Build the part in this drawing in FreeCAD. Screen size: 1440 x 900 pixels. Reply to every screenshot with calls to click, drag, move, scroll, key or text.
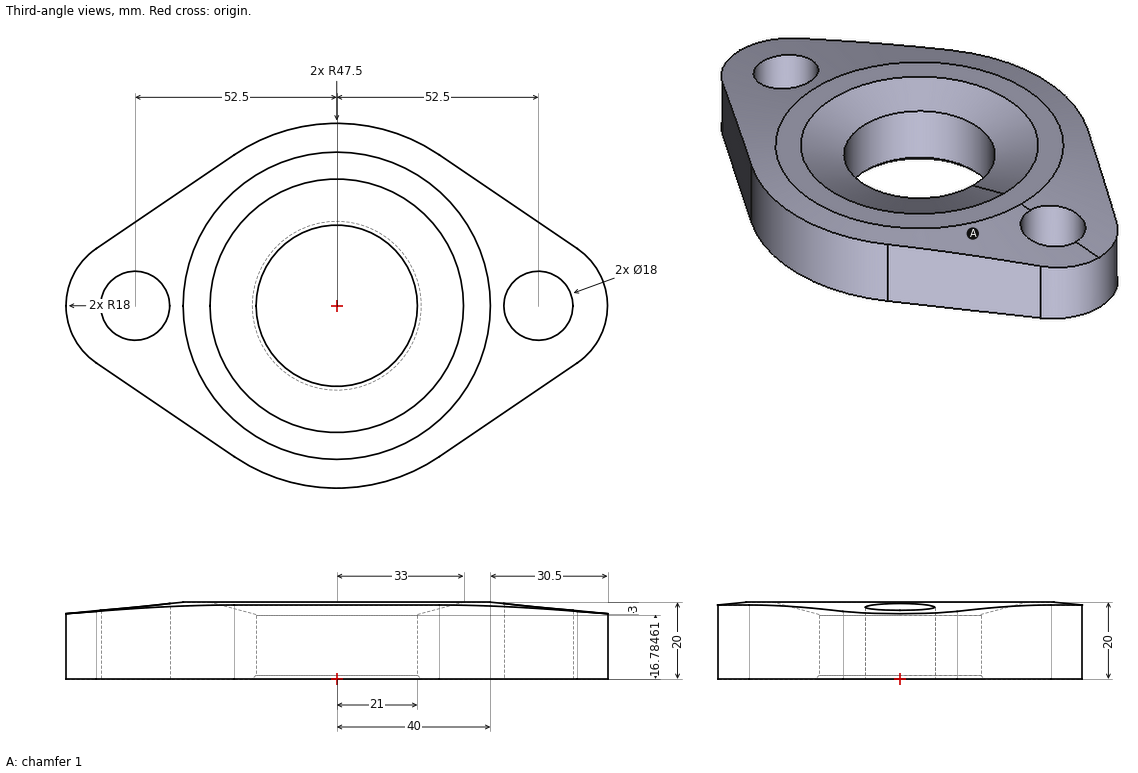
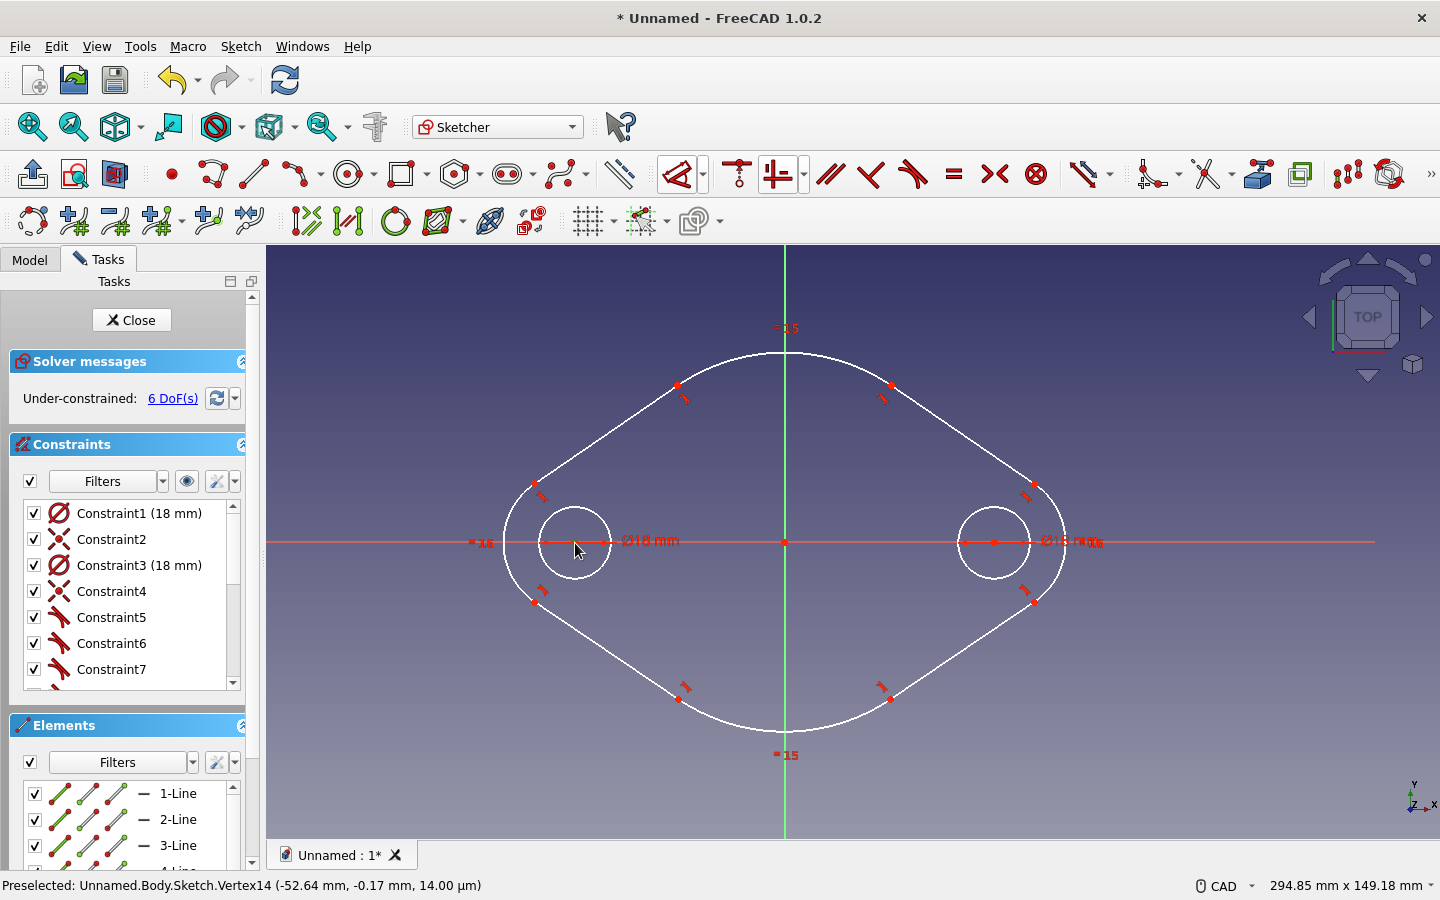
click(364, 542)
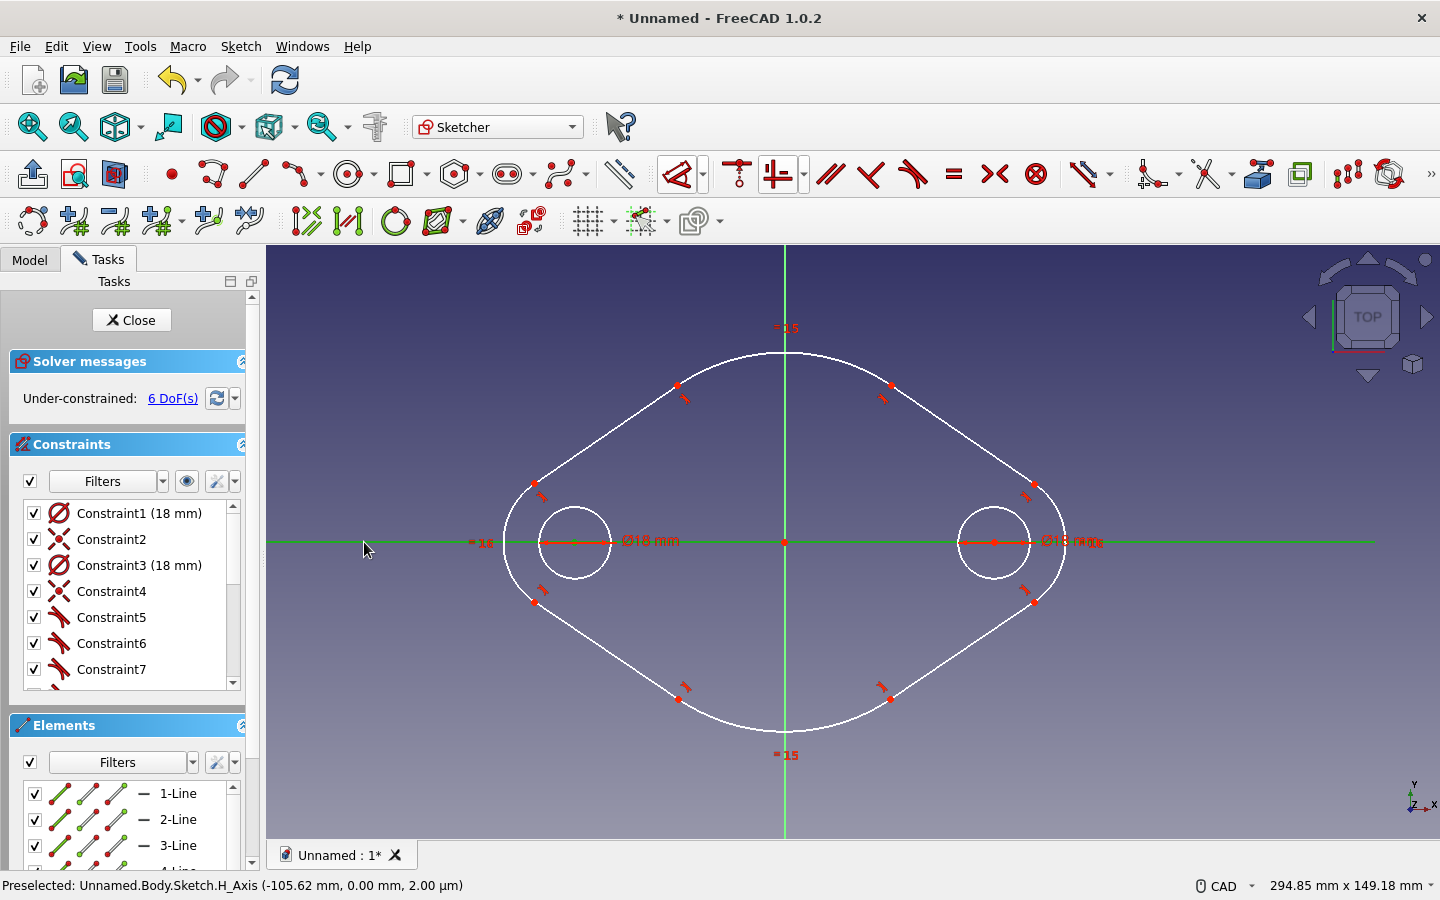
click(737, 174)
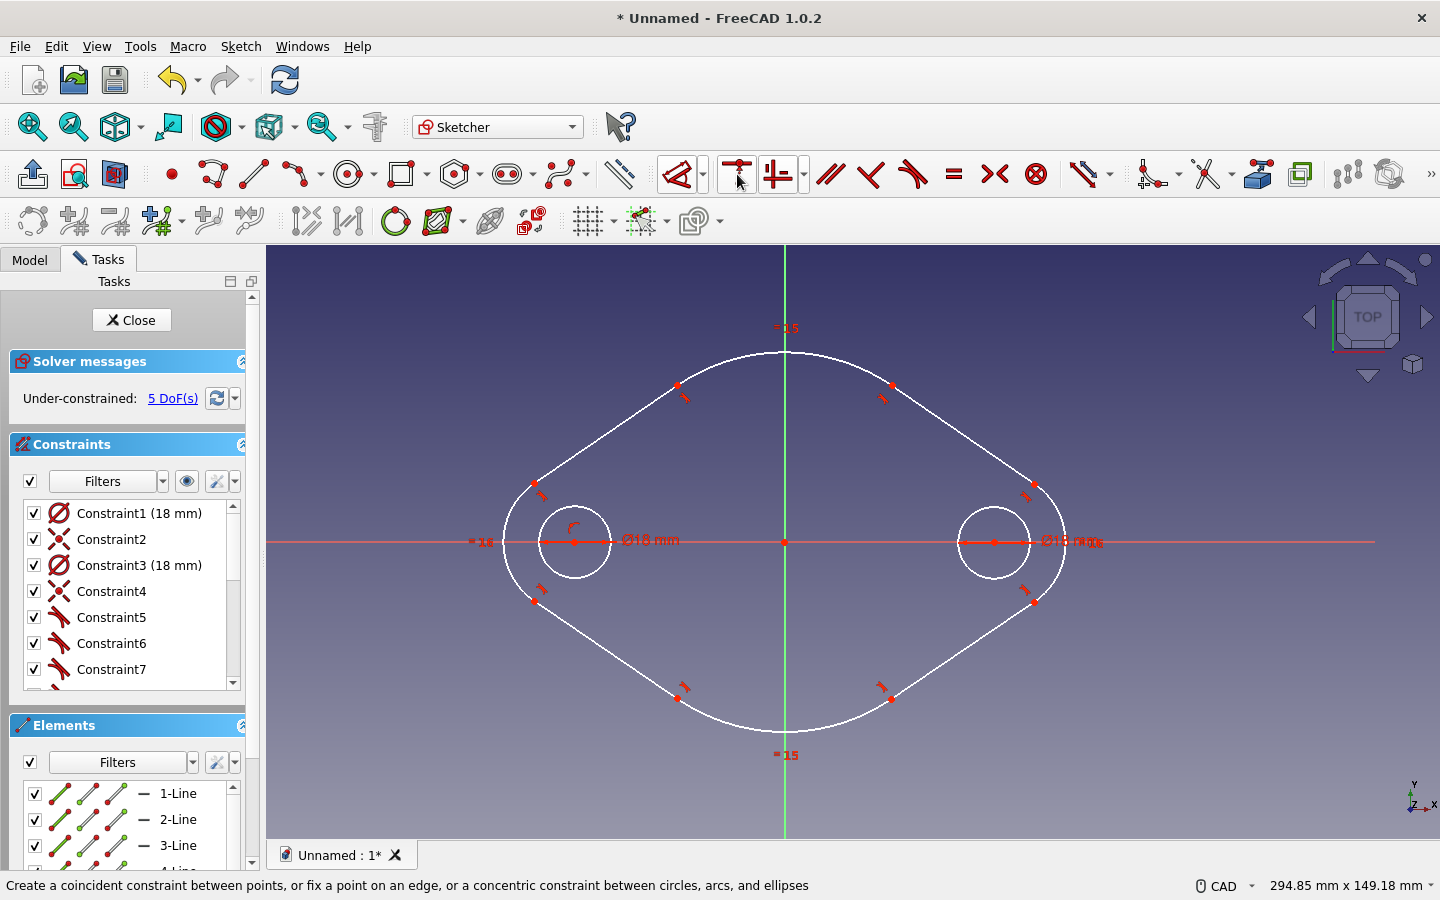
click(994, 543)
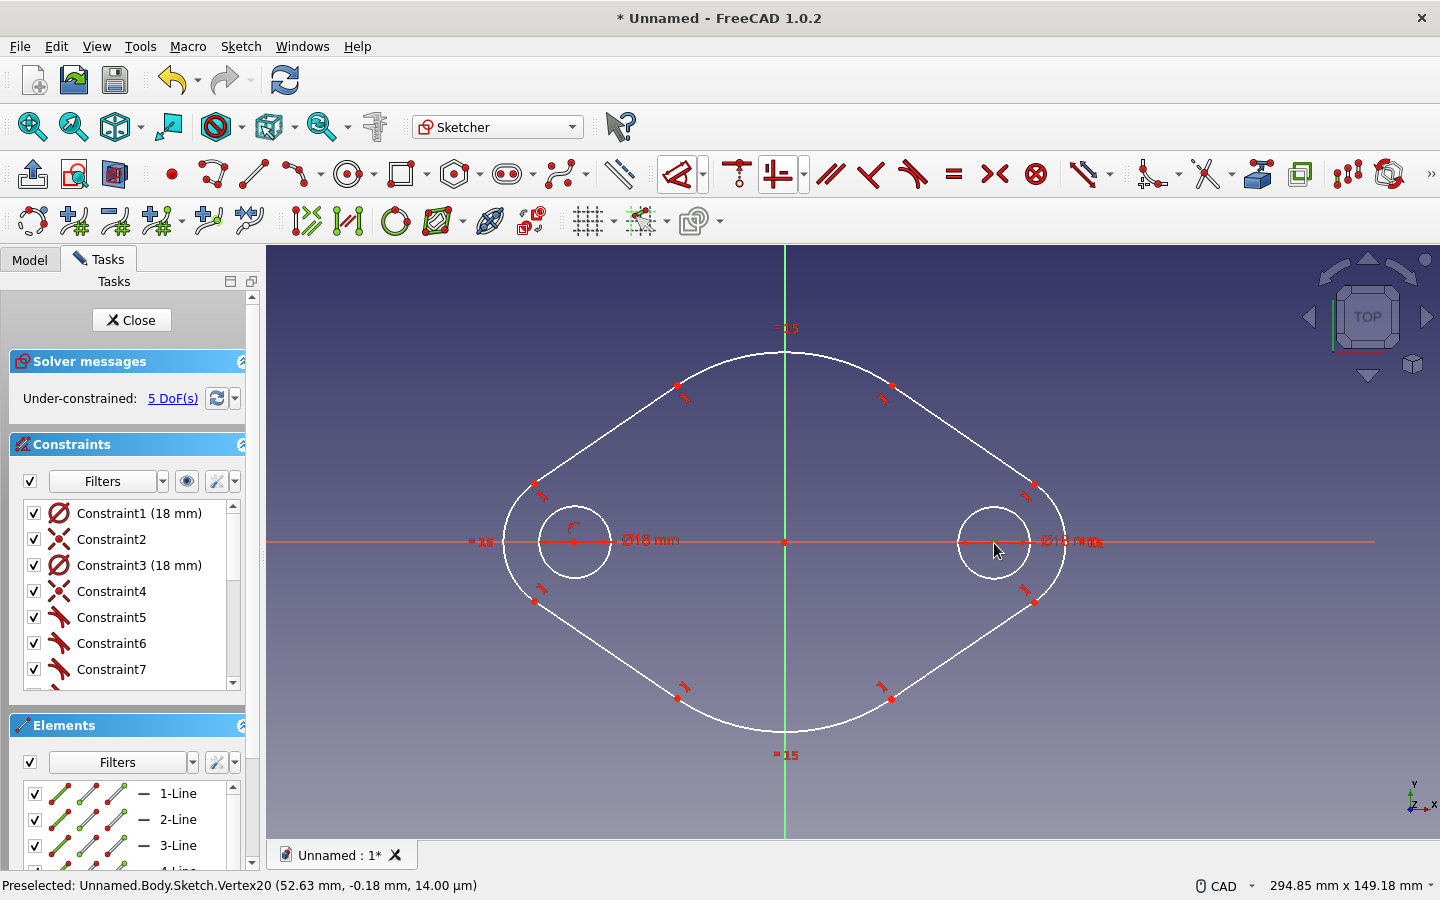
click(364, 542)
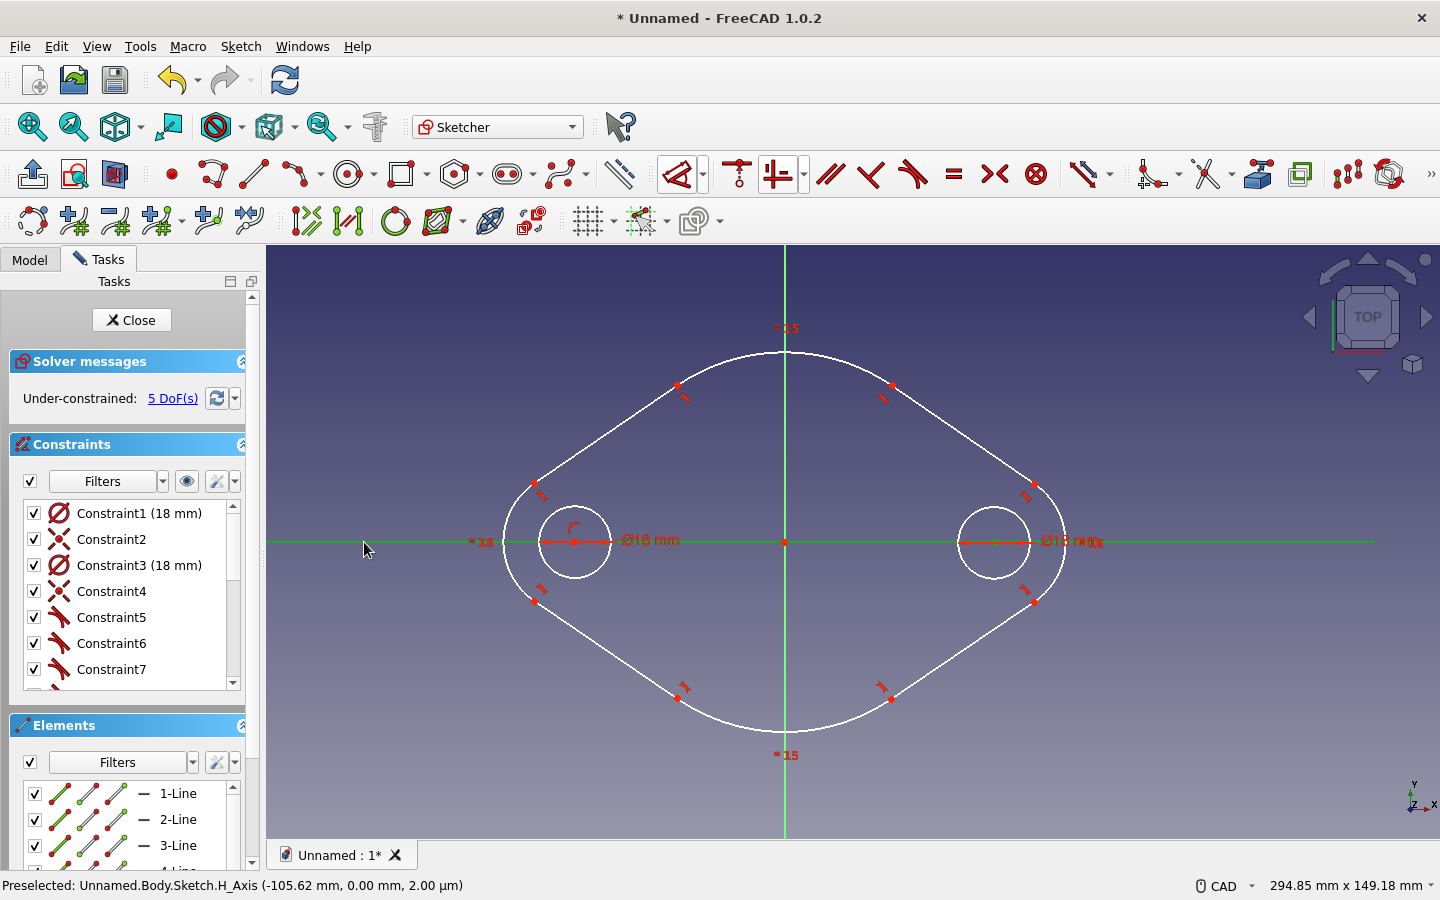
key(c)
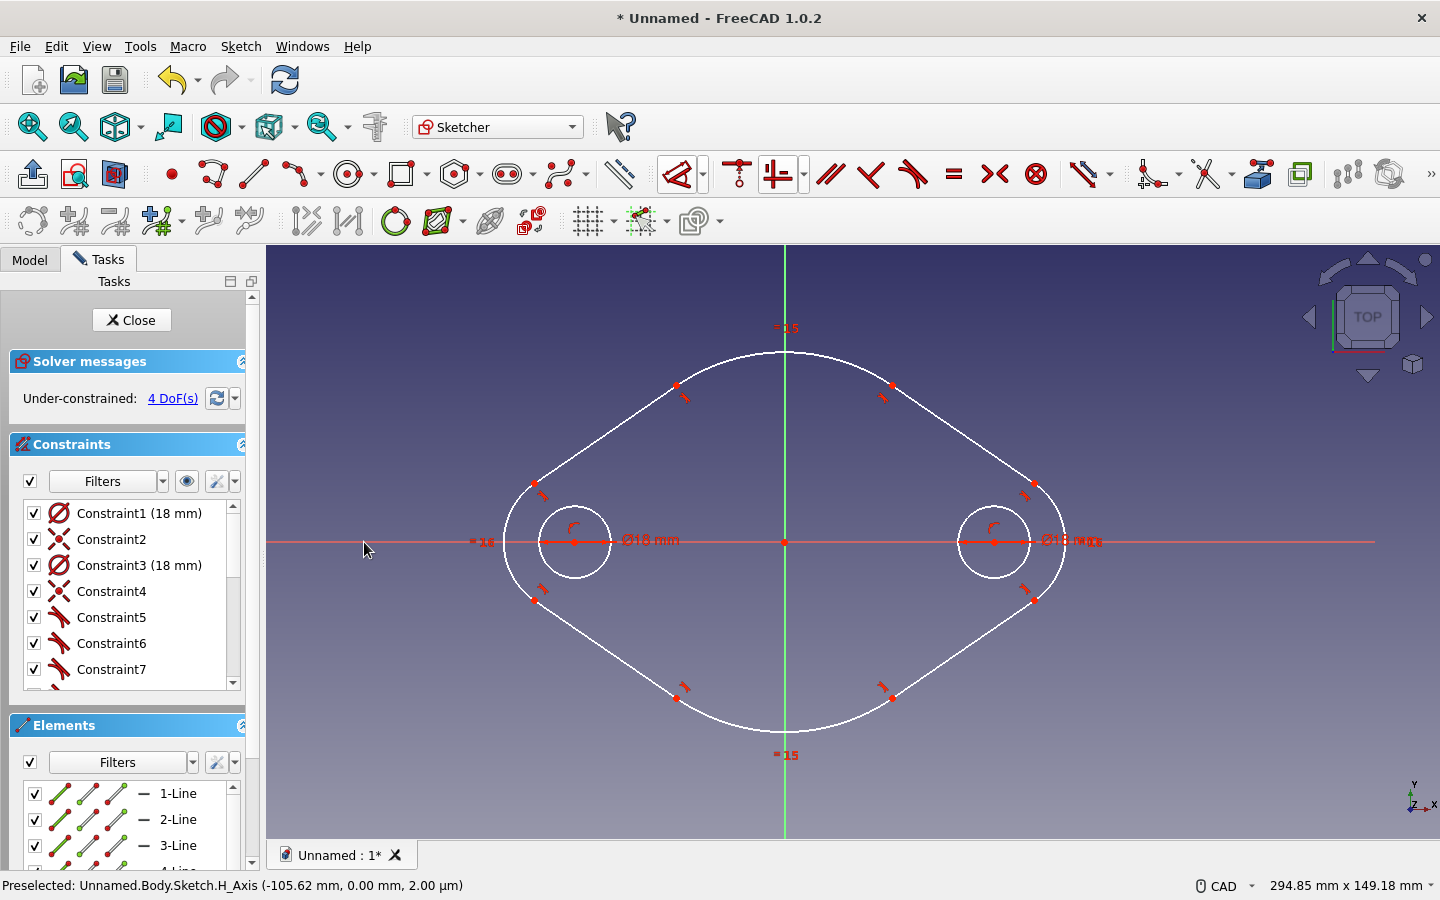
key(d)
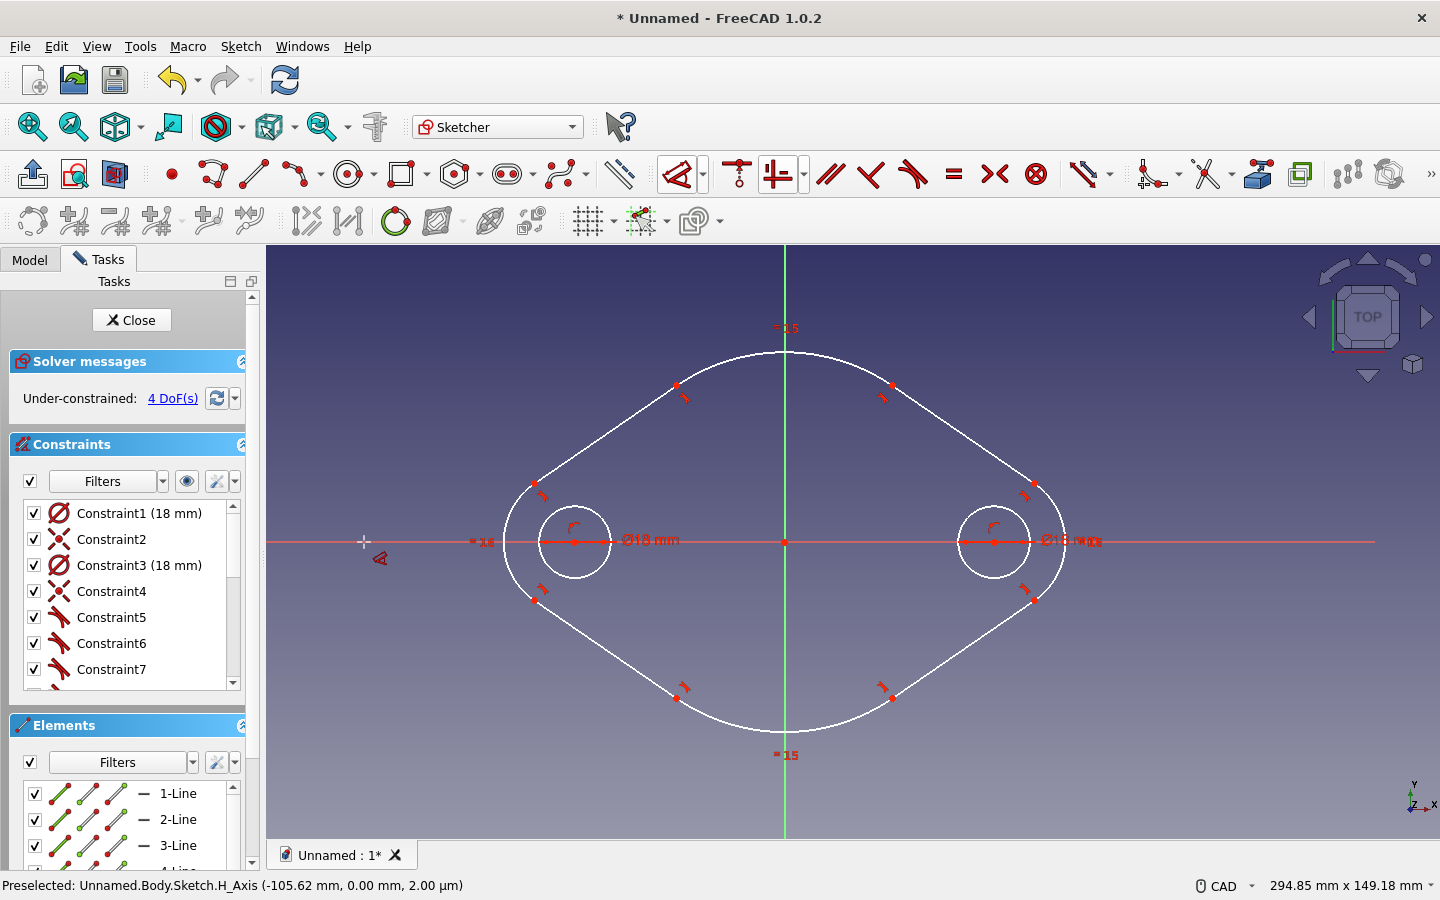
click(830, 358)
click(838, 327)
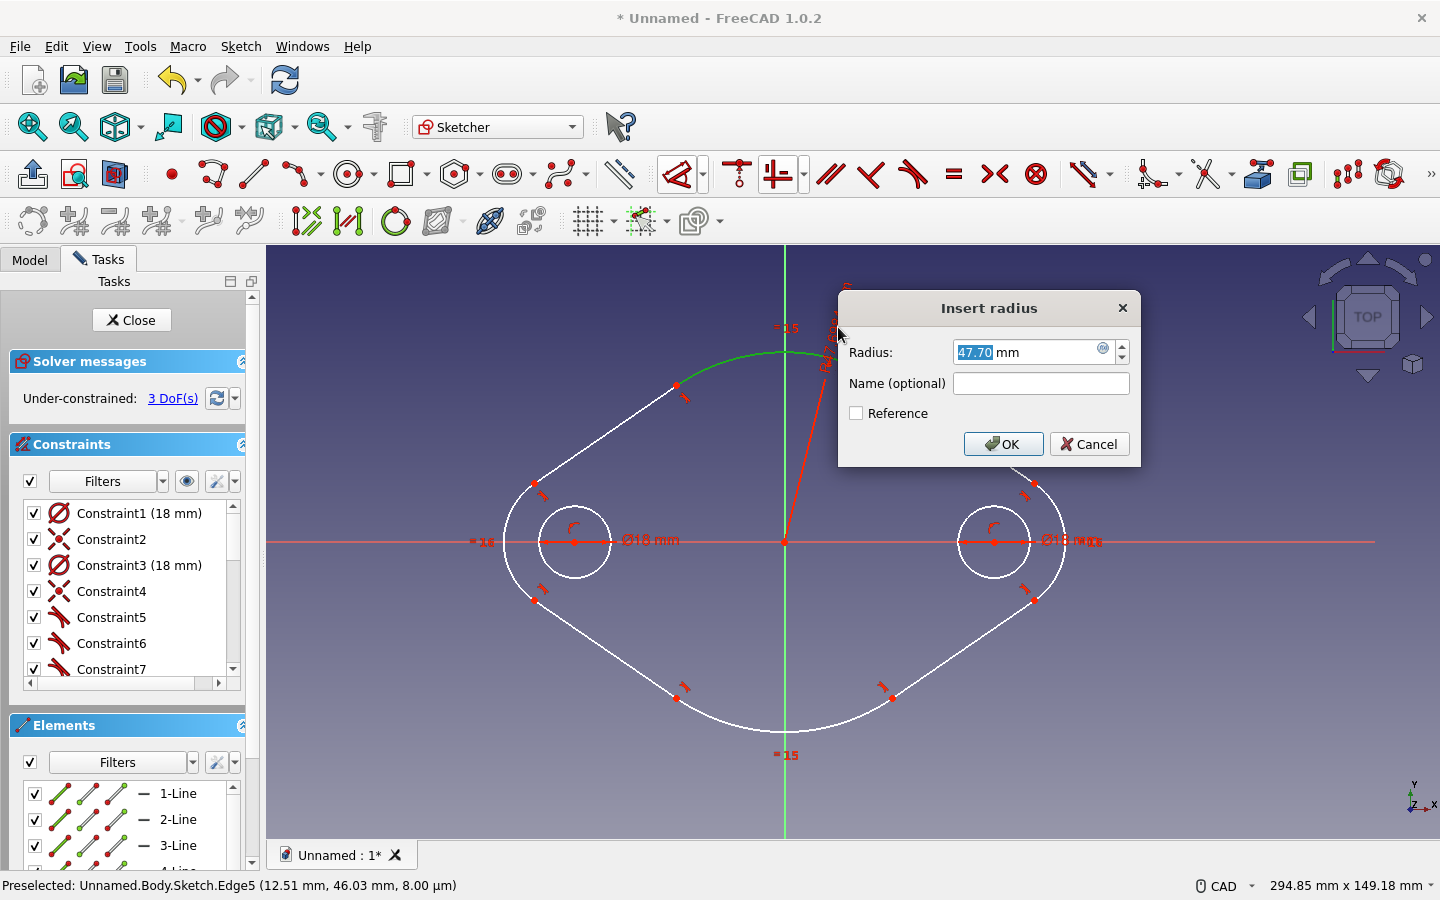
text(47.5)
key(Return)